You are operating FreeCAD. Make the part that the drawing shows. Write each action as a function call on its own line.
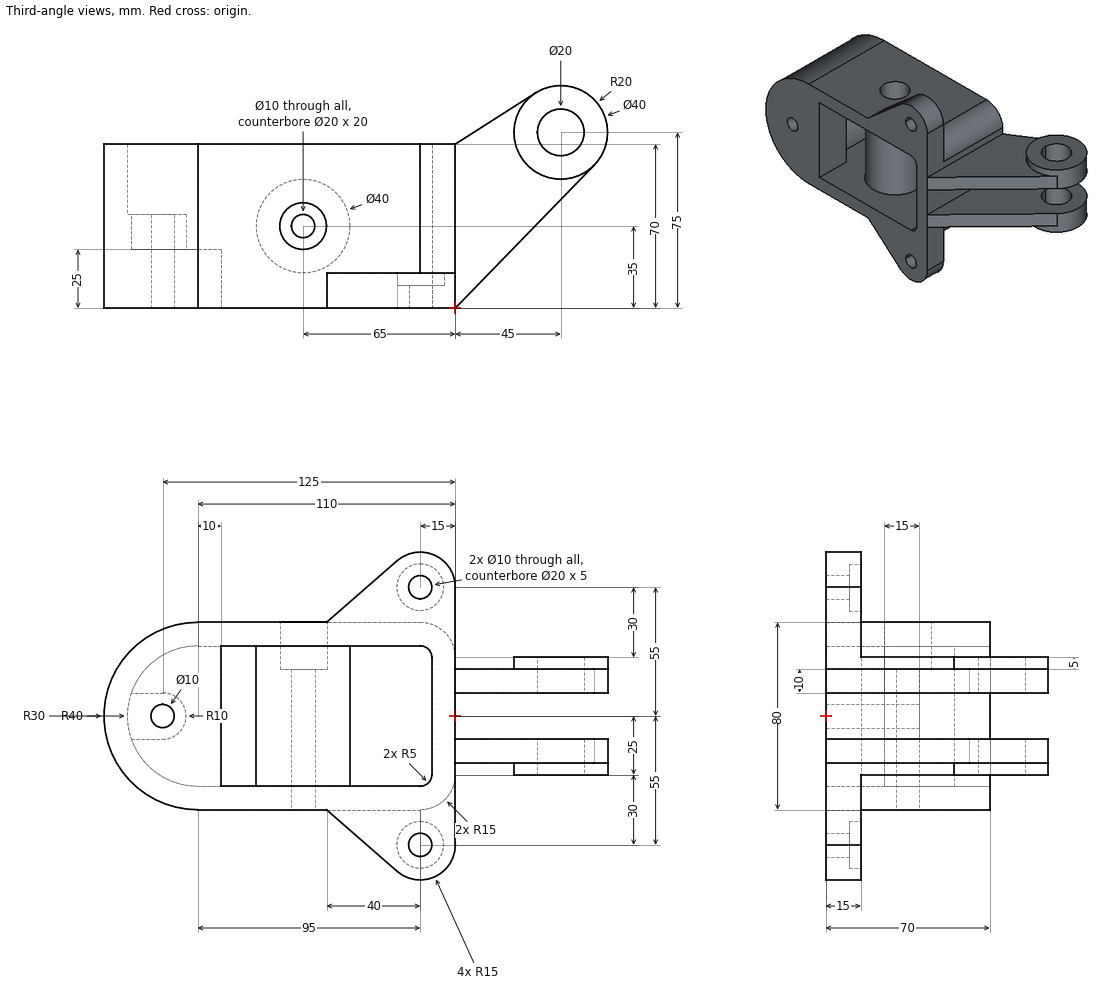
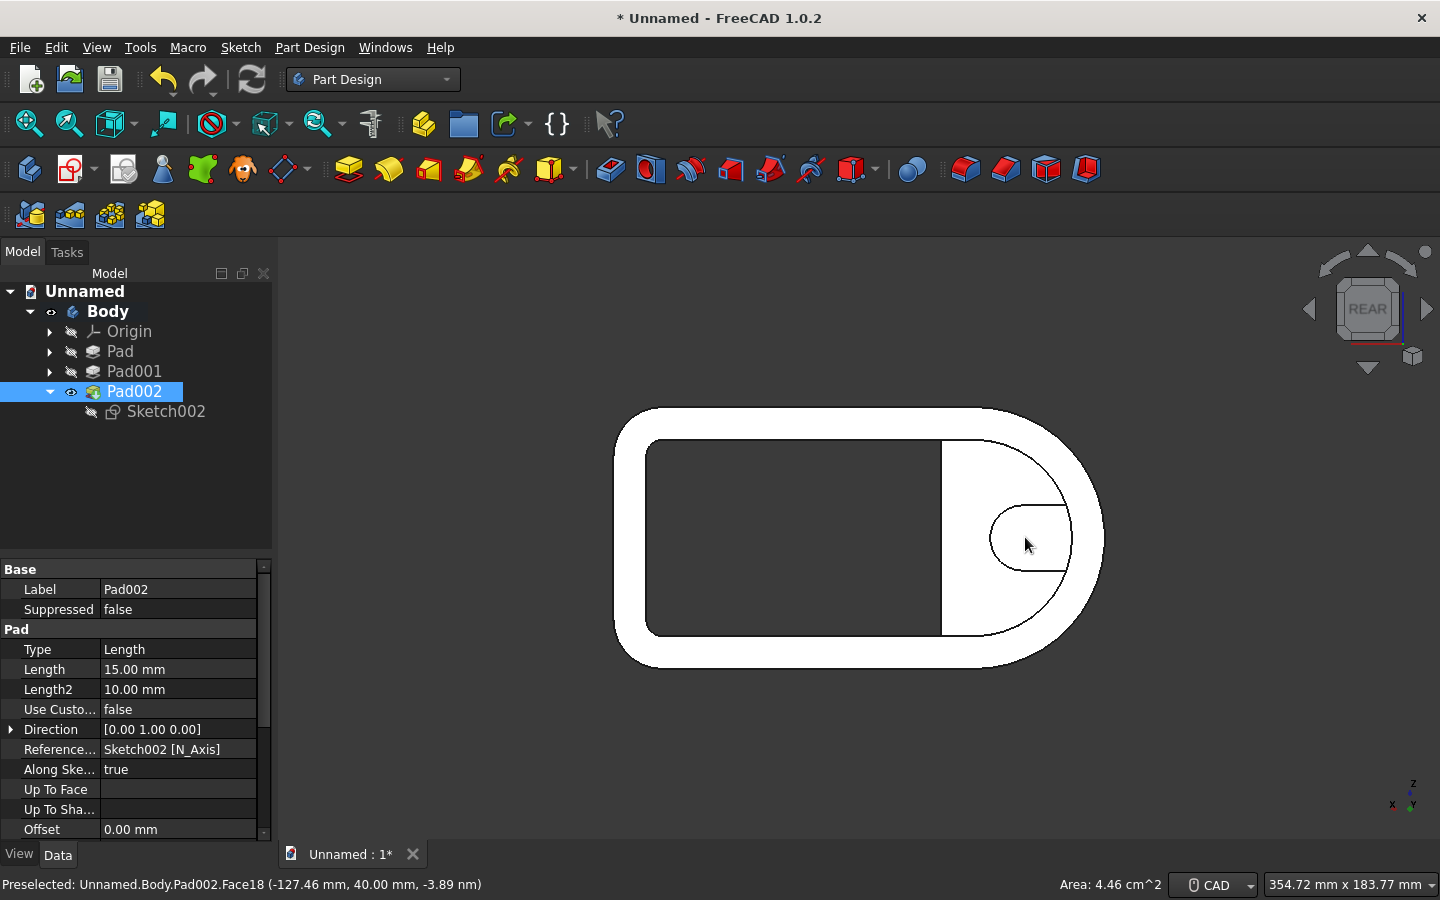
click(70, 170)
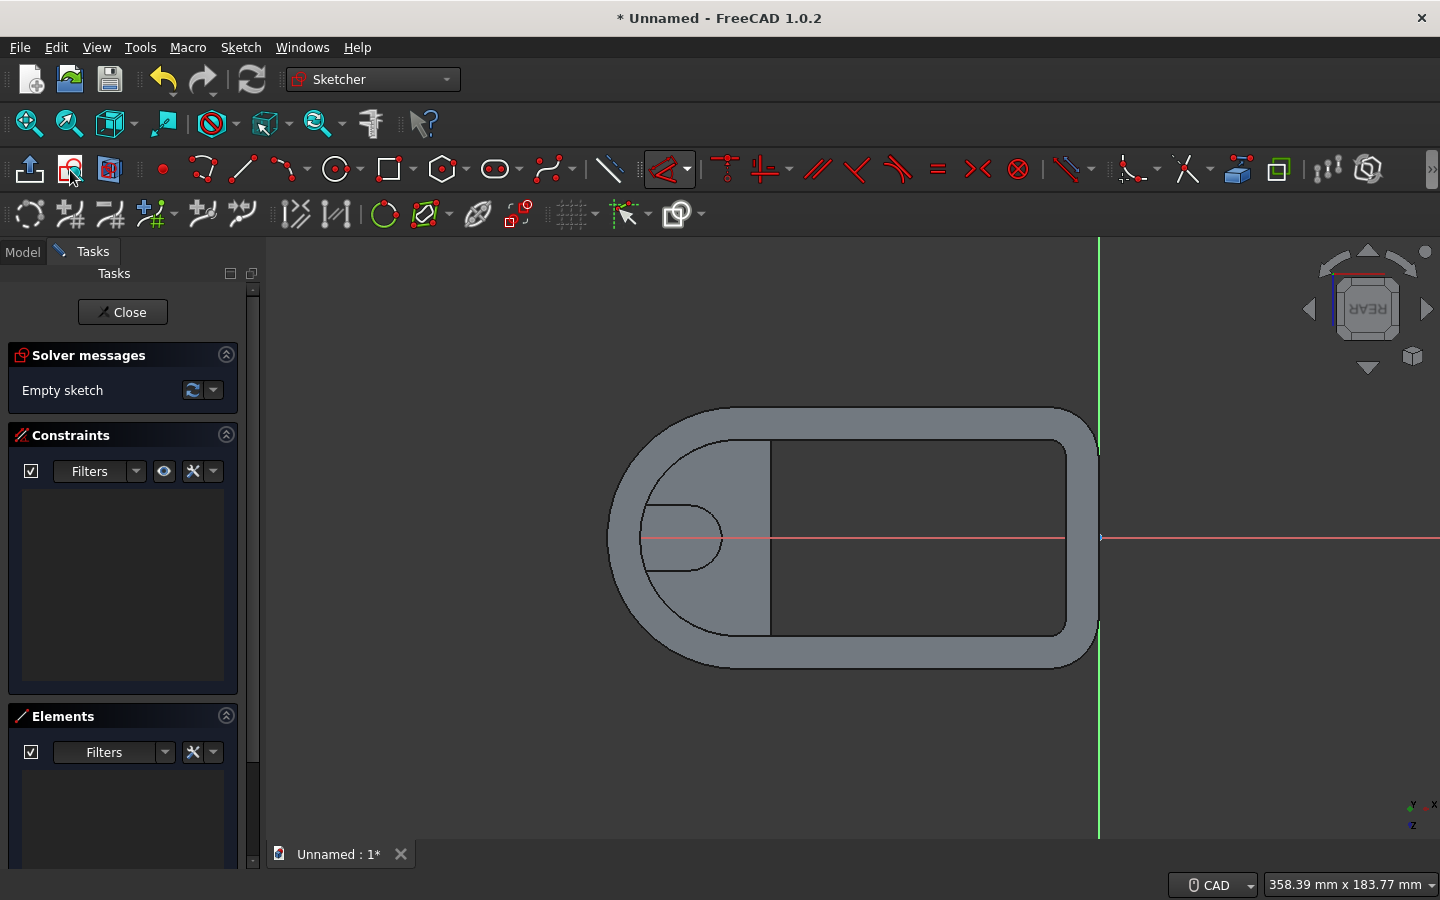
click(110, 170)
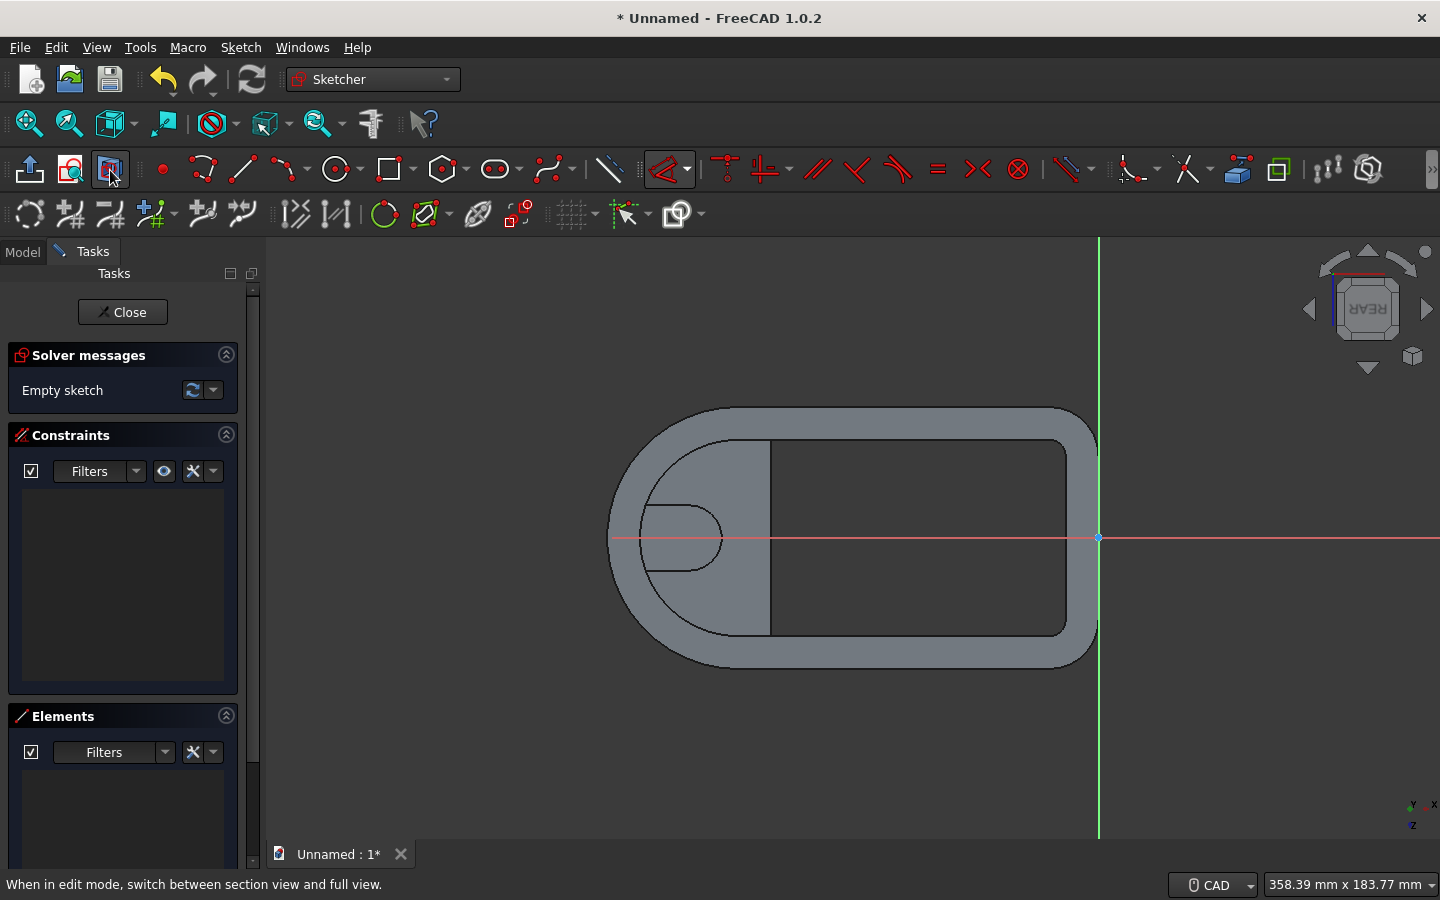
scroll(680, 538, up, 12)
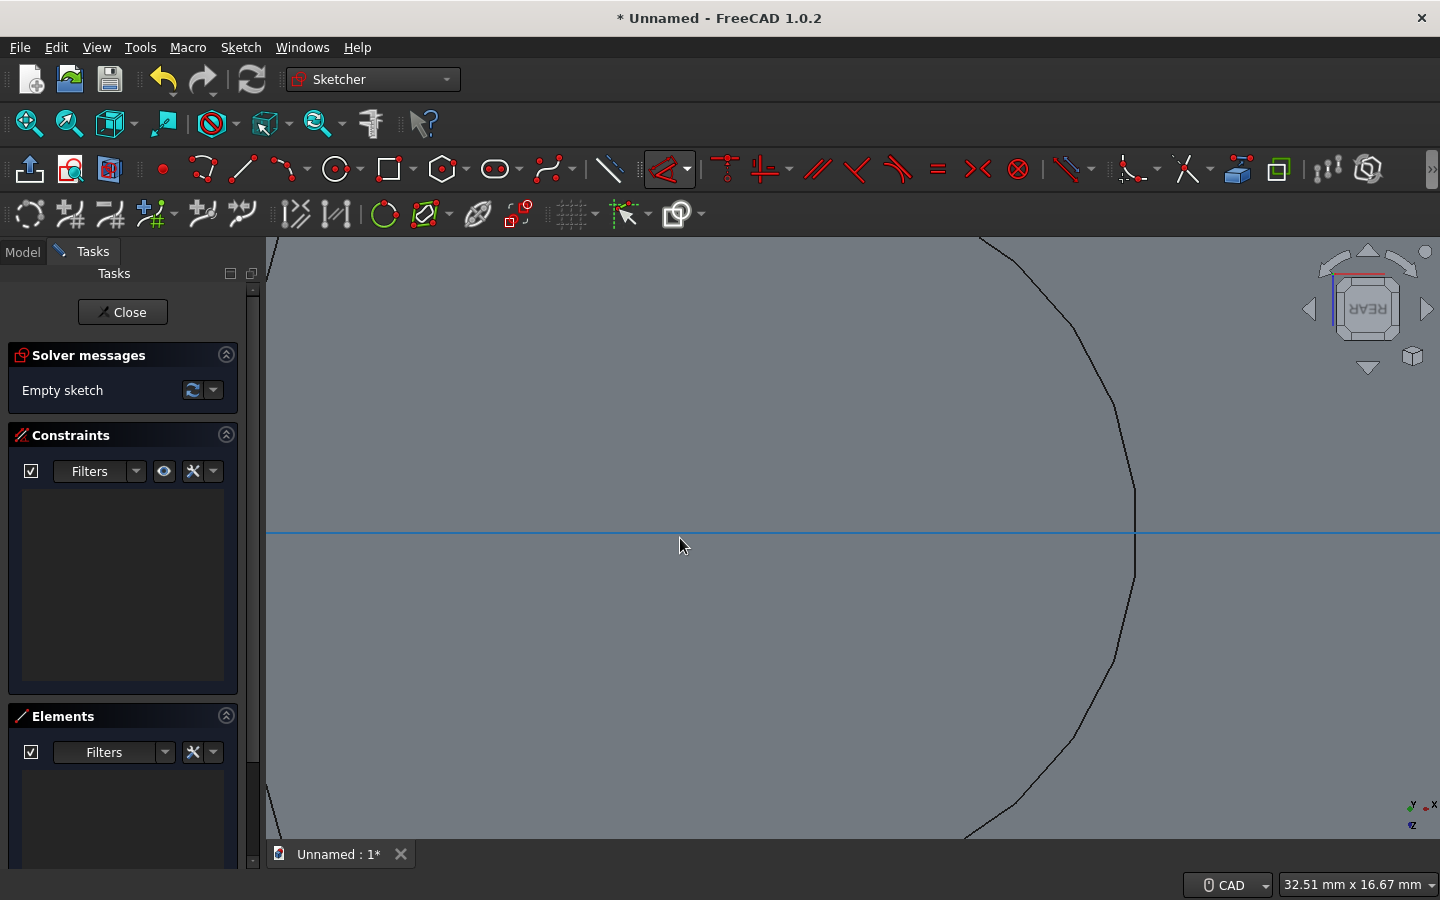
key(g)
key(c)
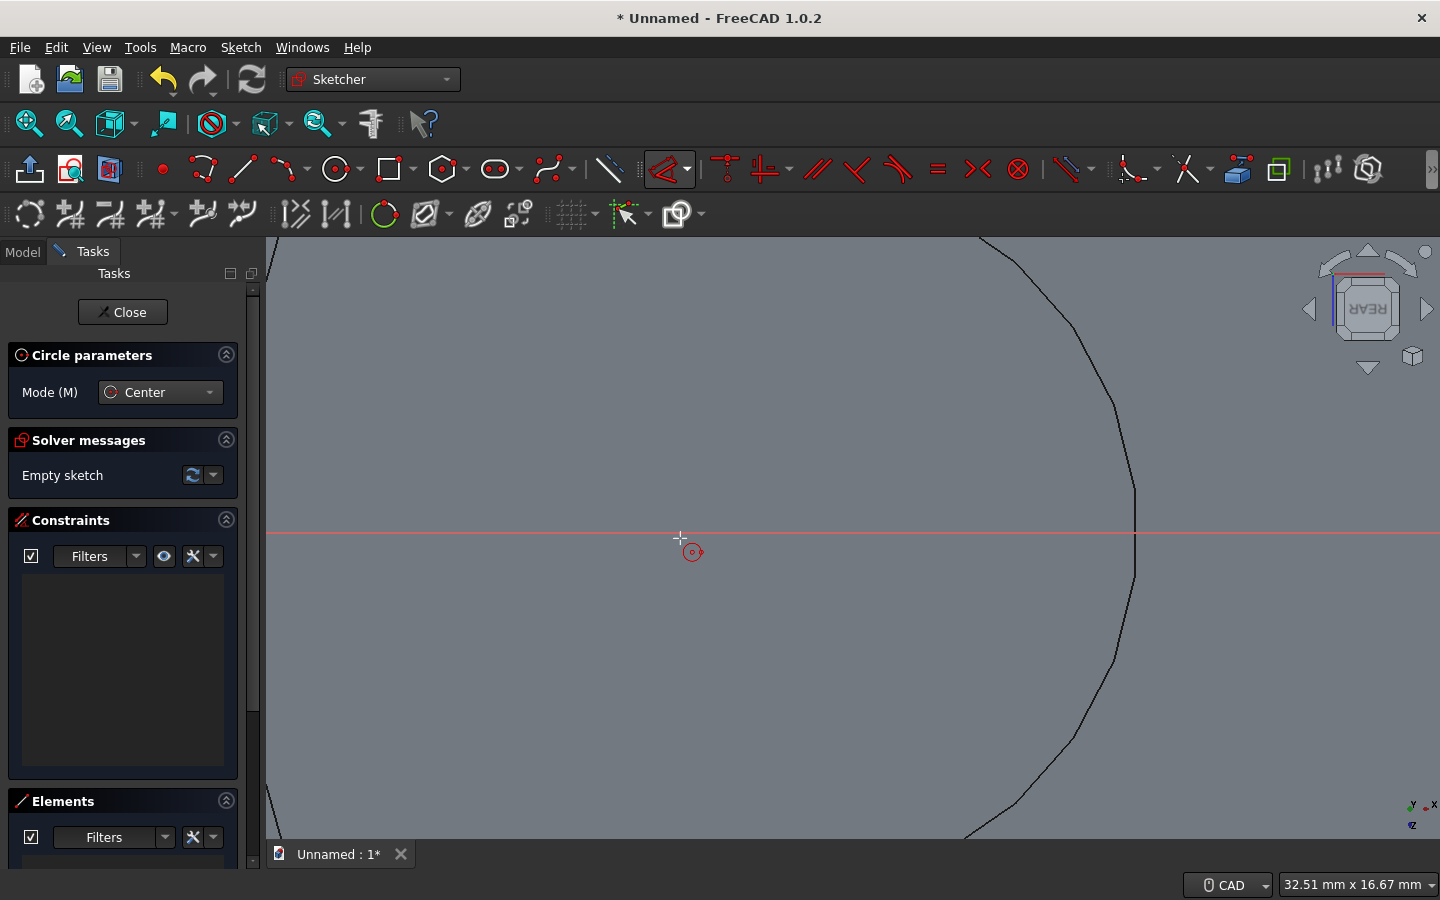
click(776, 533)
move(904, 405)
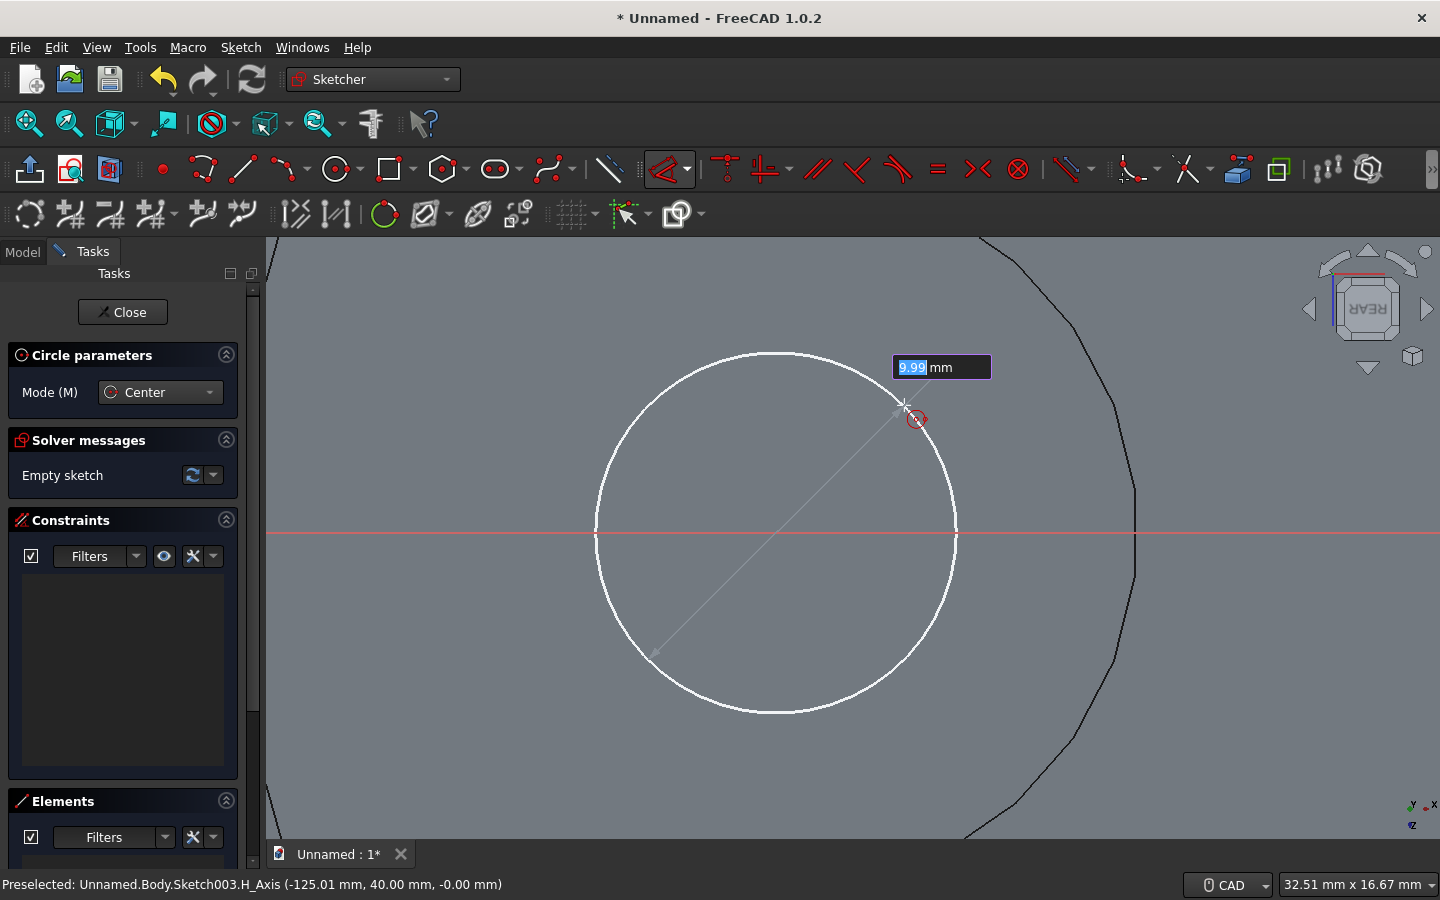
text(10)
key(Return)
key(Escape)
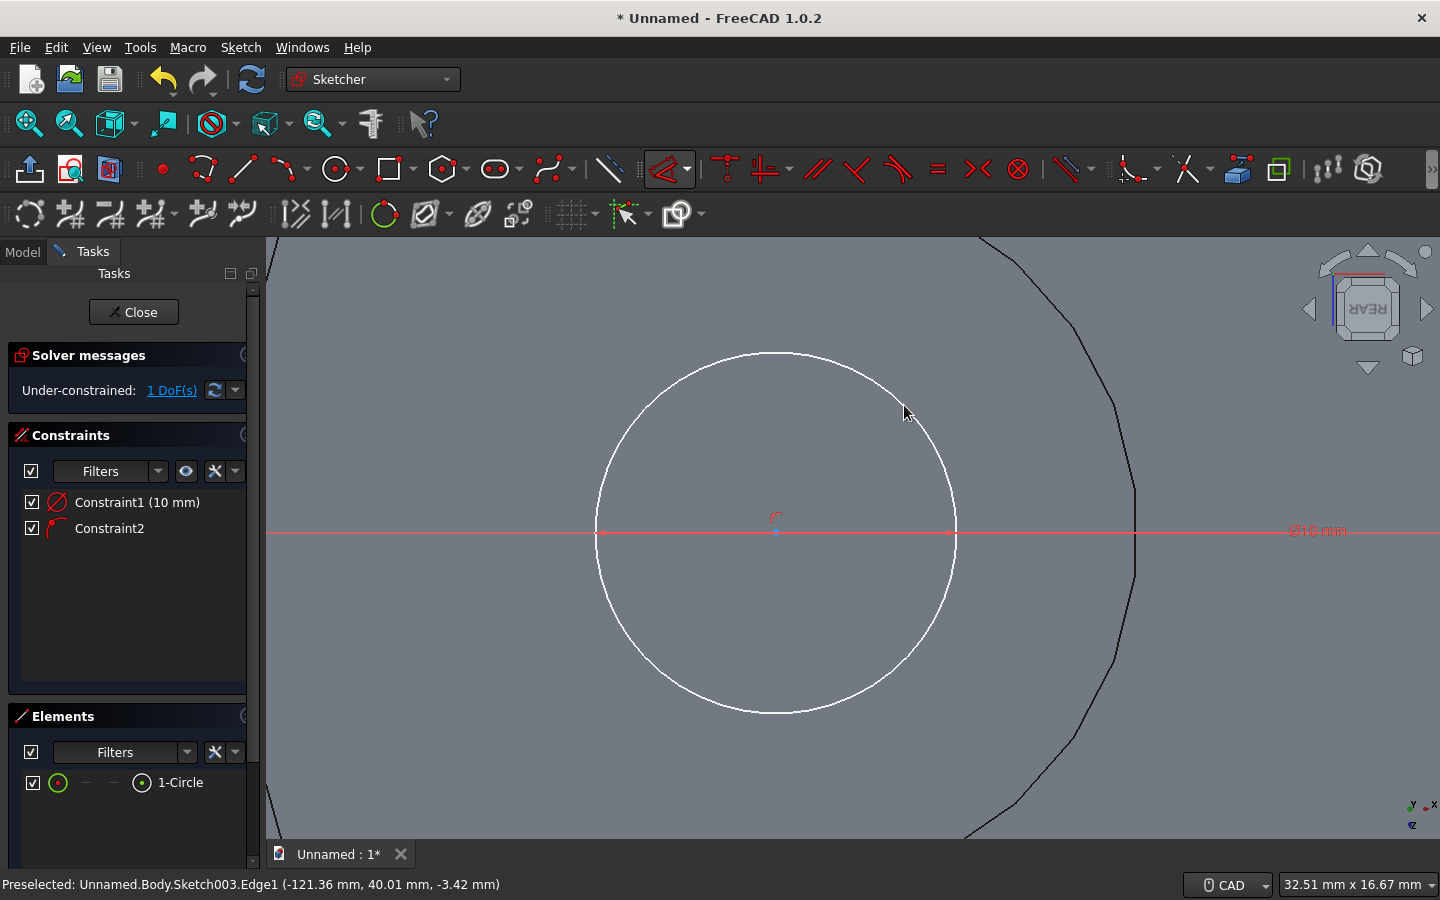
click(776, 533)